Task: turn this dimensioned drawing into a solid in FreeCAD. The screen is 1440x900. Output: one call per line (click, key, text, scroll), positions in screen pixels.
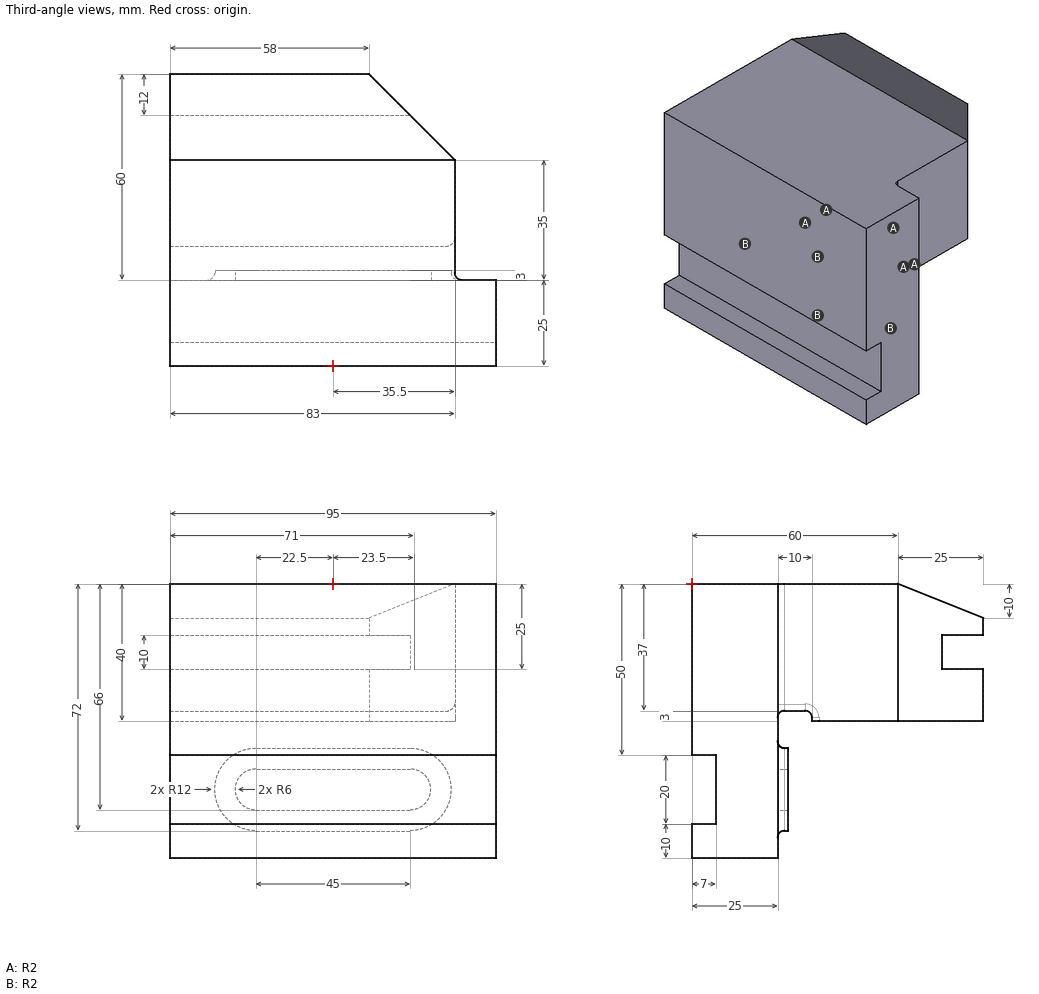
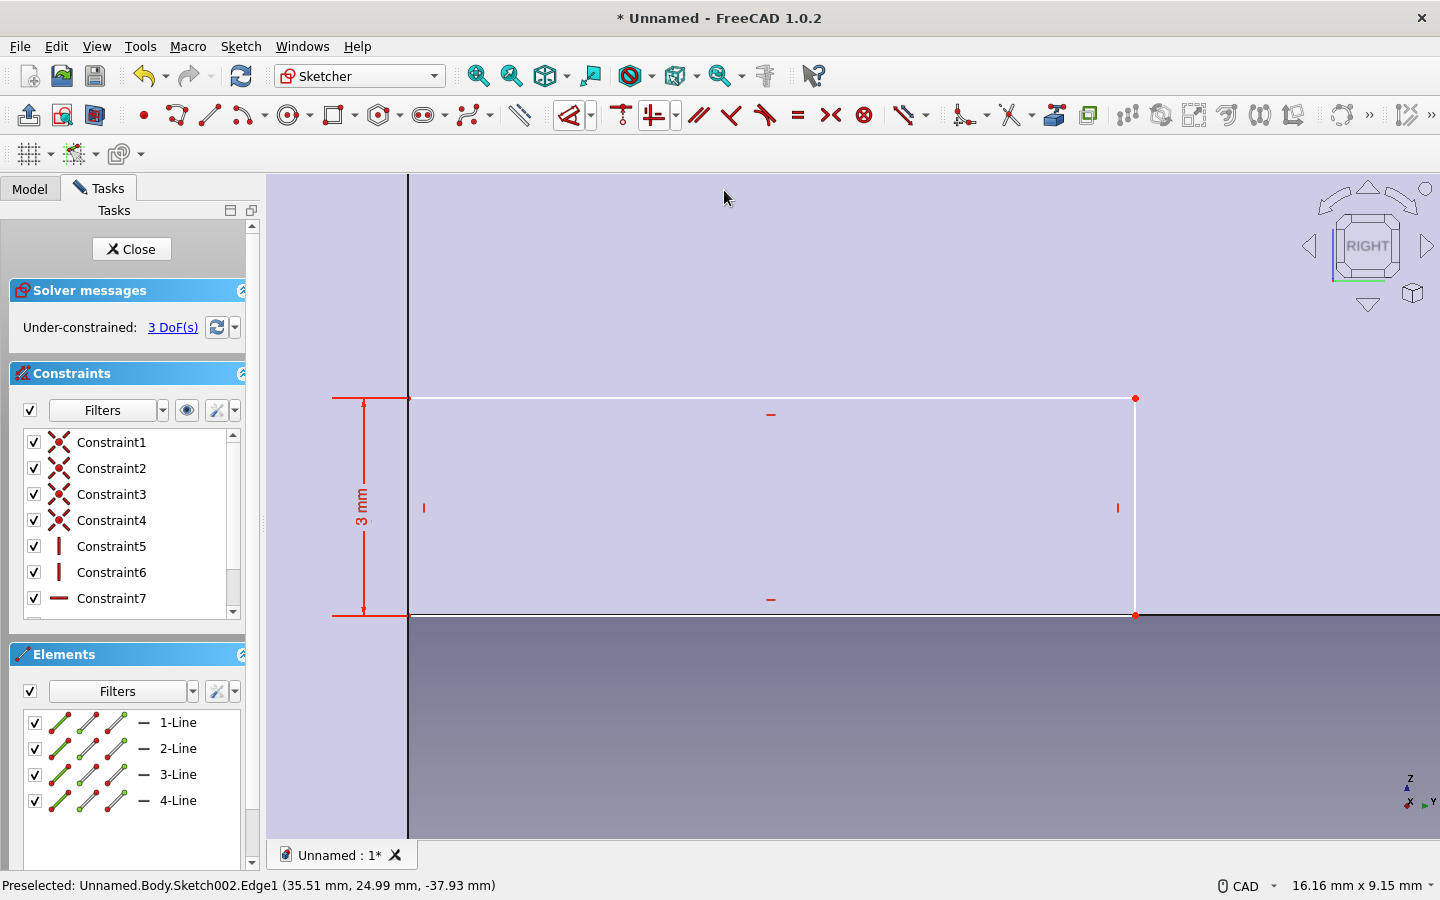
click(626, 616)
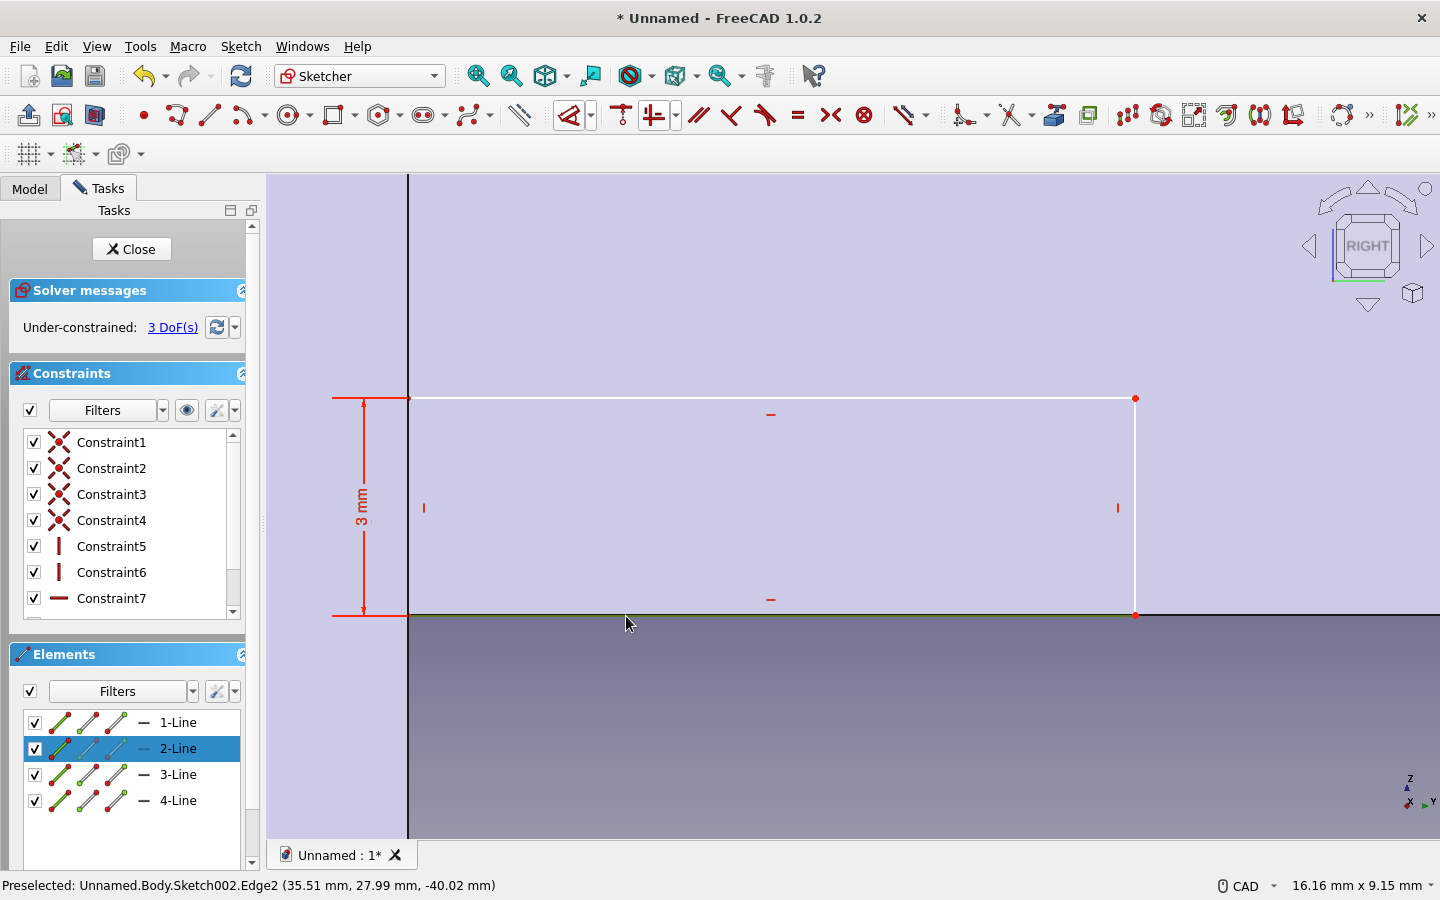
key(l)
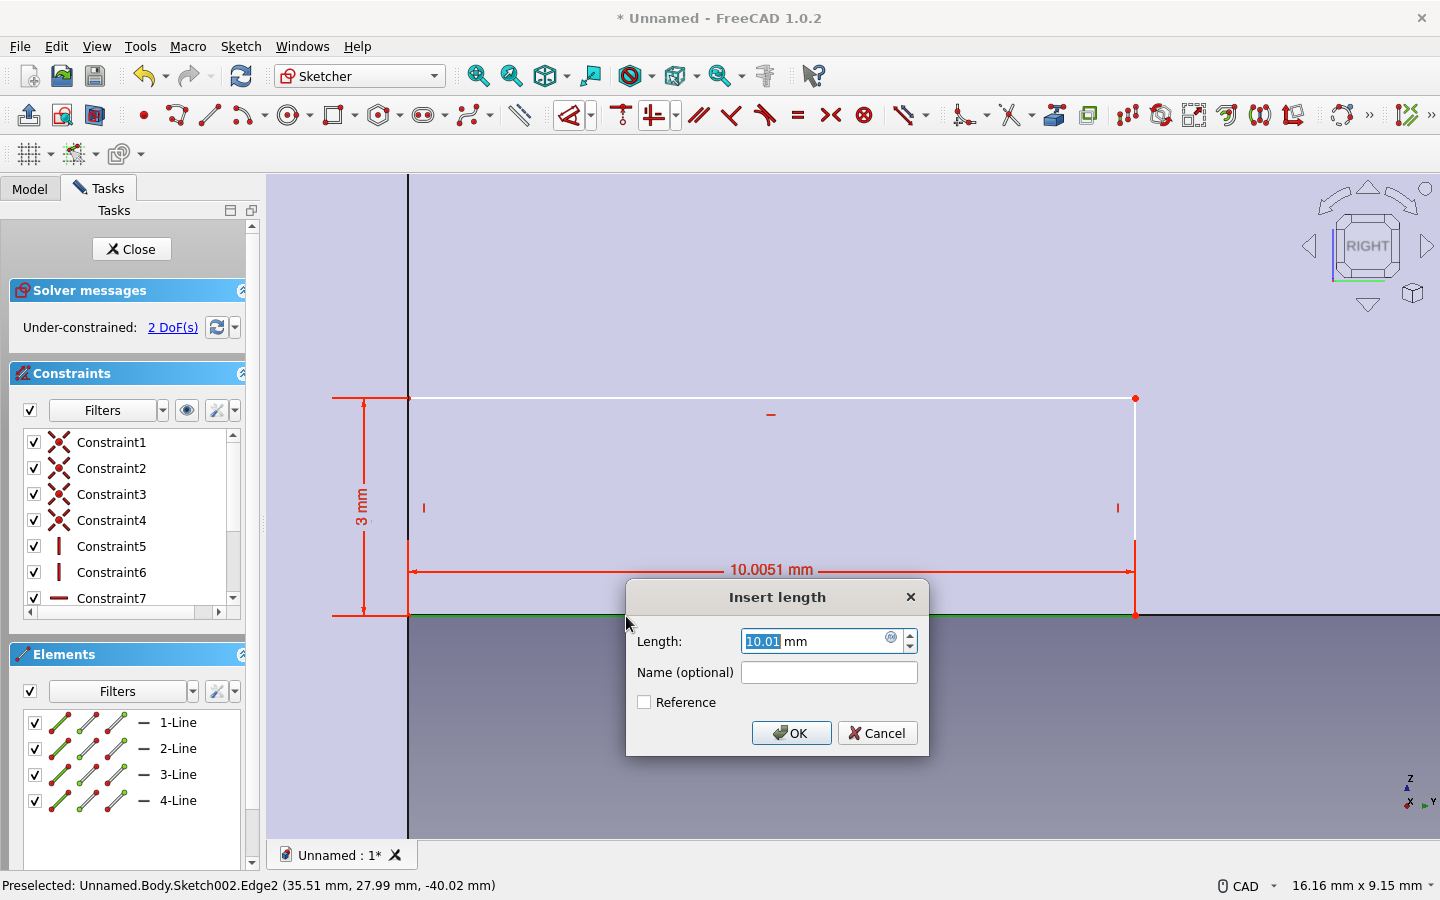
text(10)
key(Return)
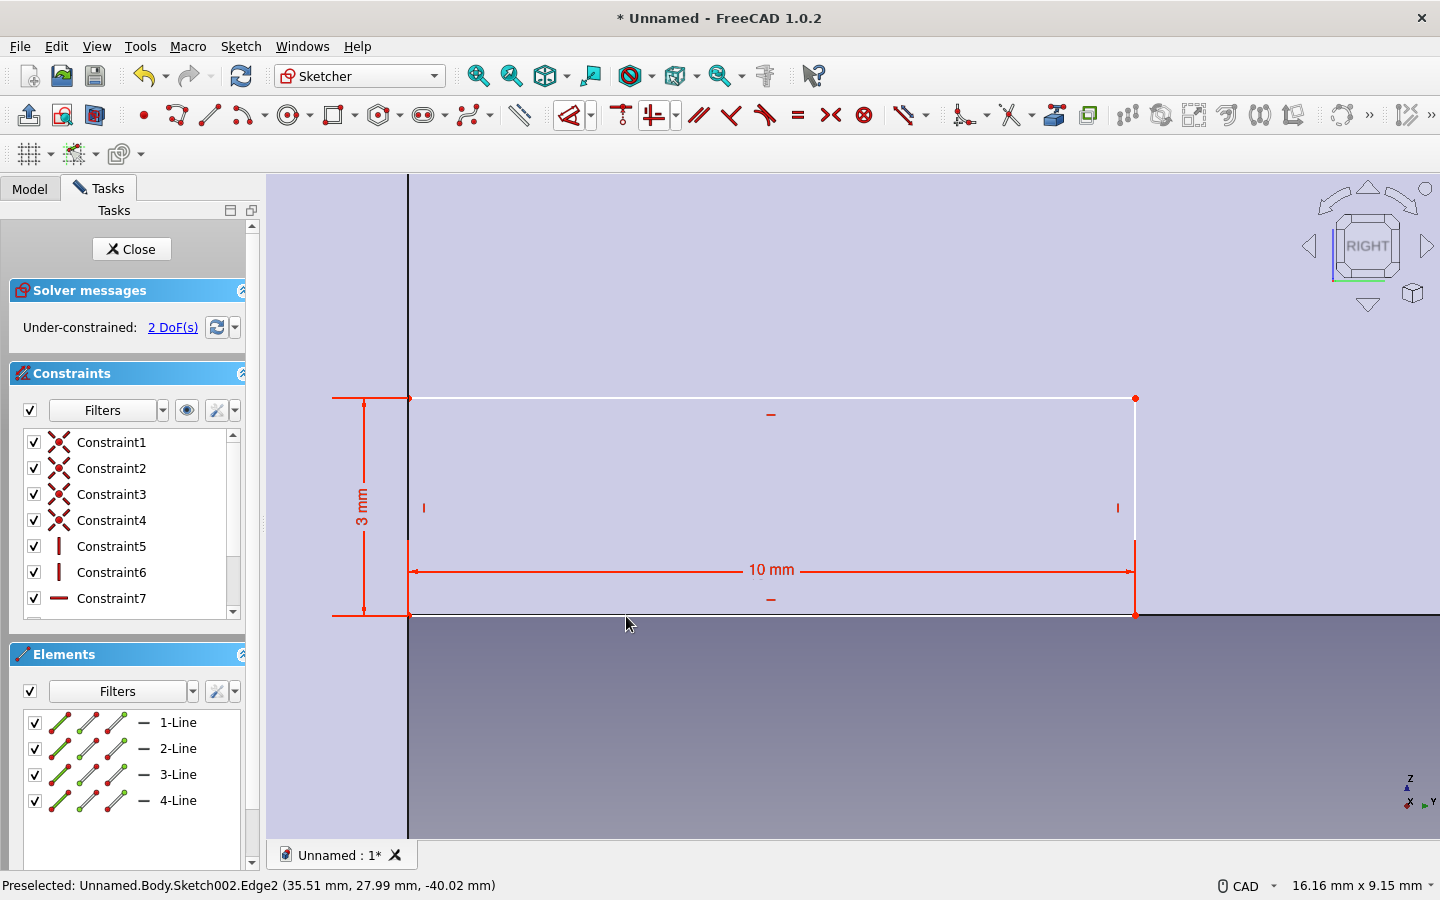
click(408, 398)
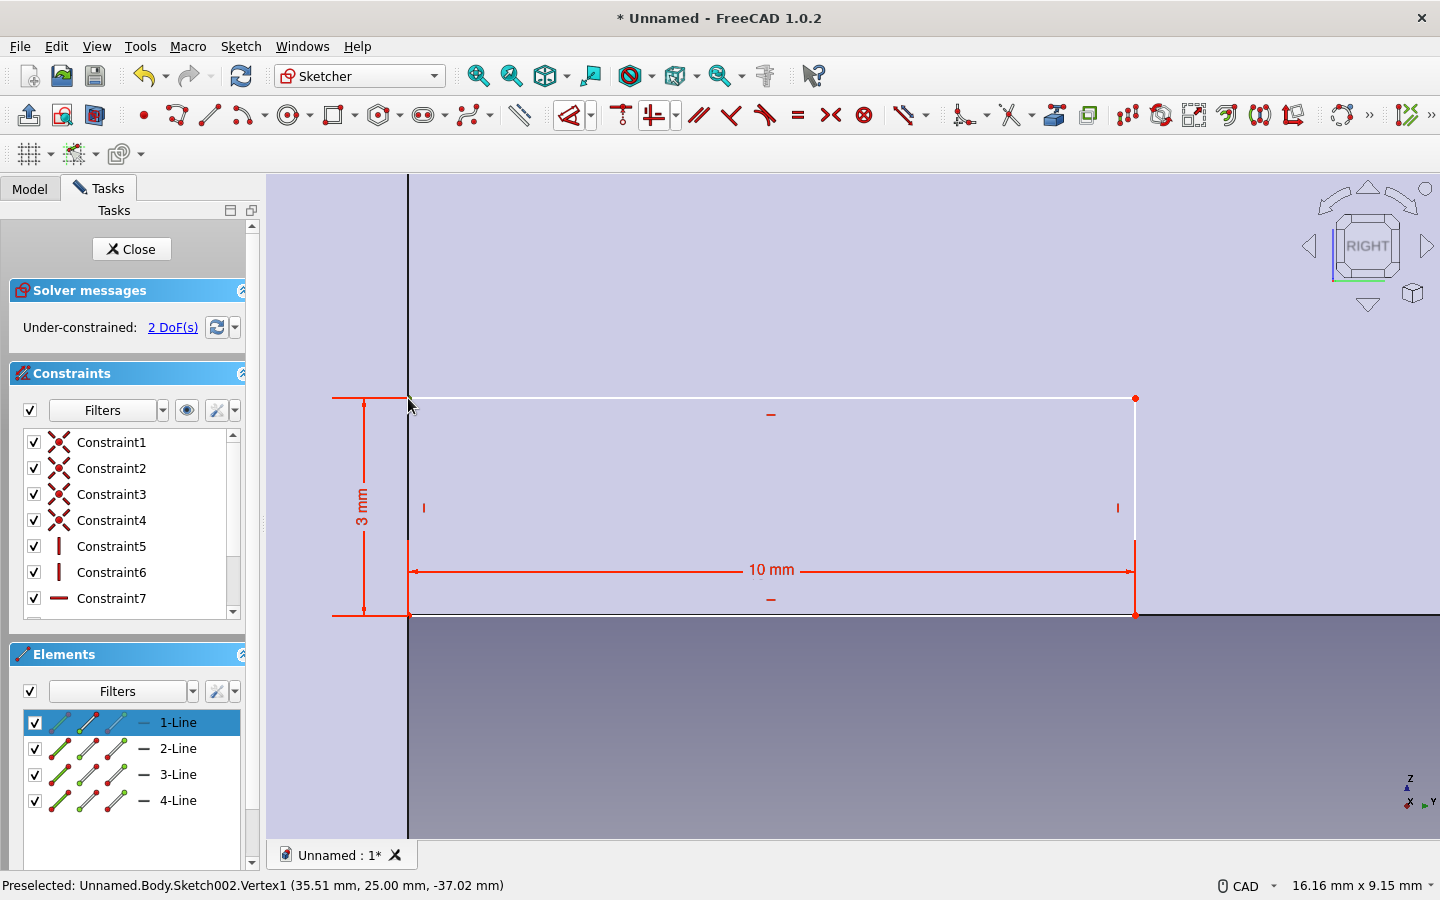
key(l)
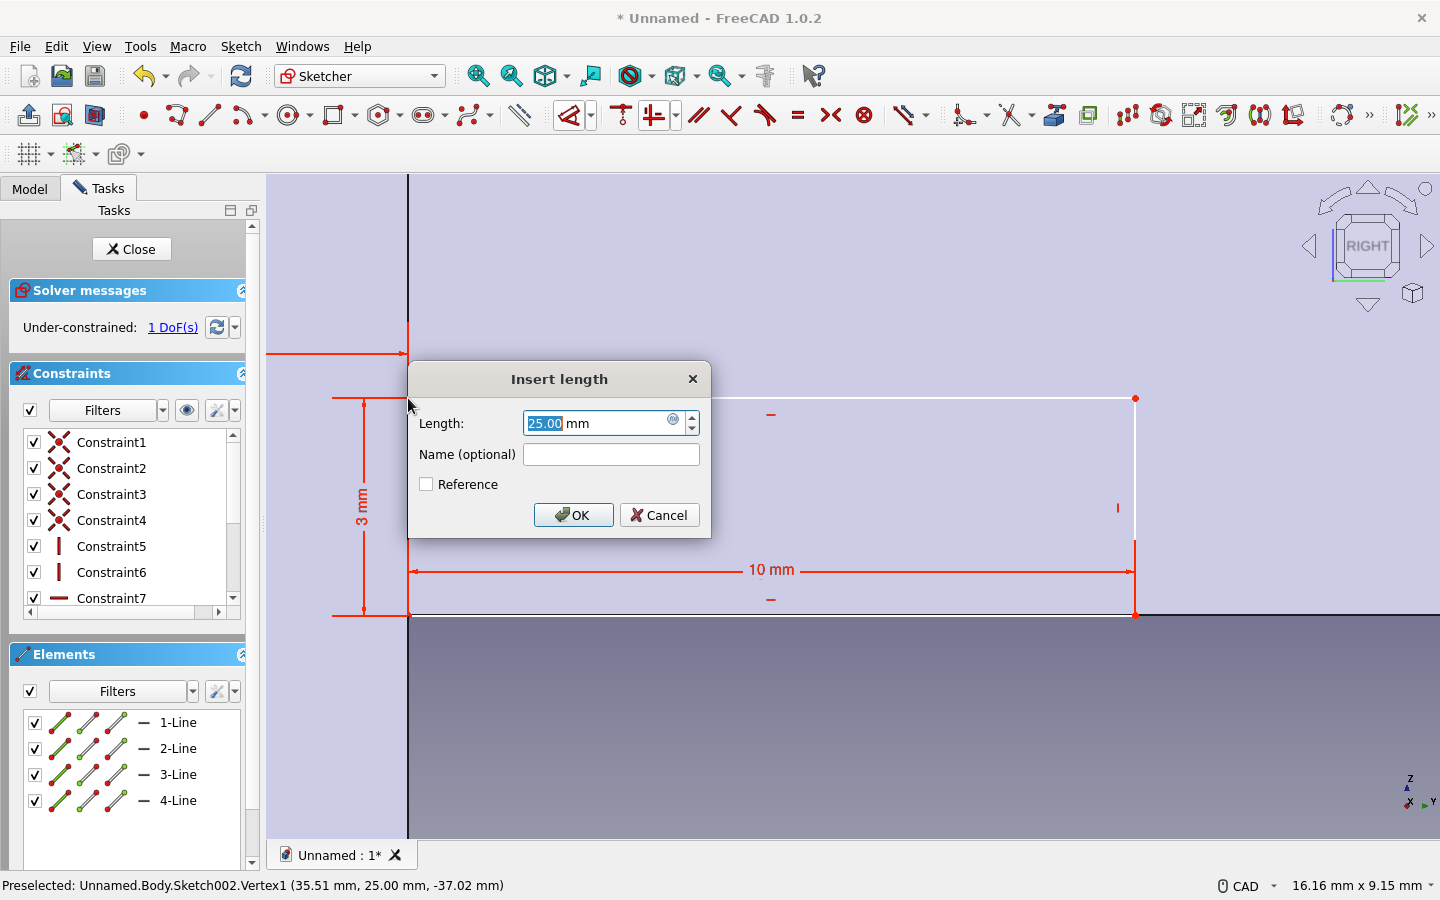
text(25)
key(Return)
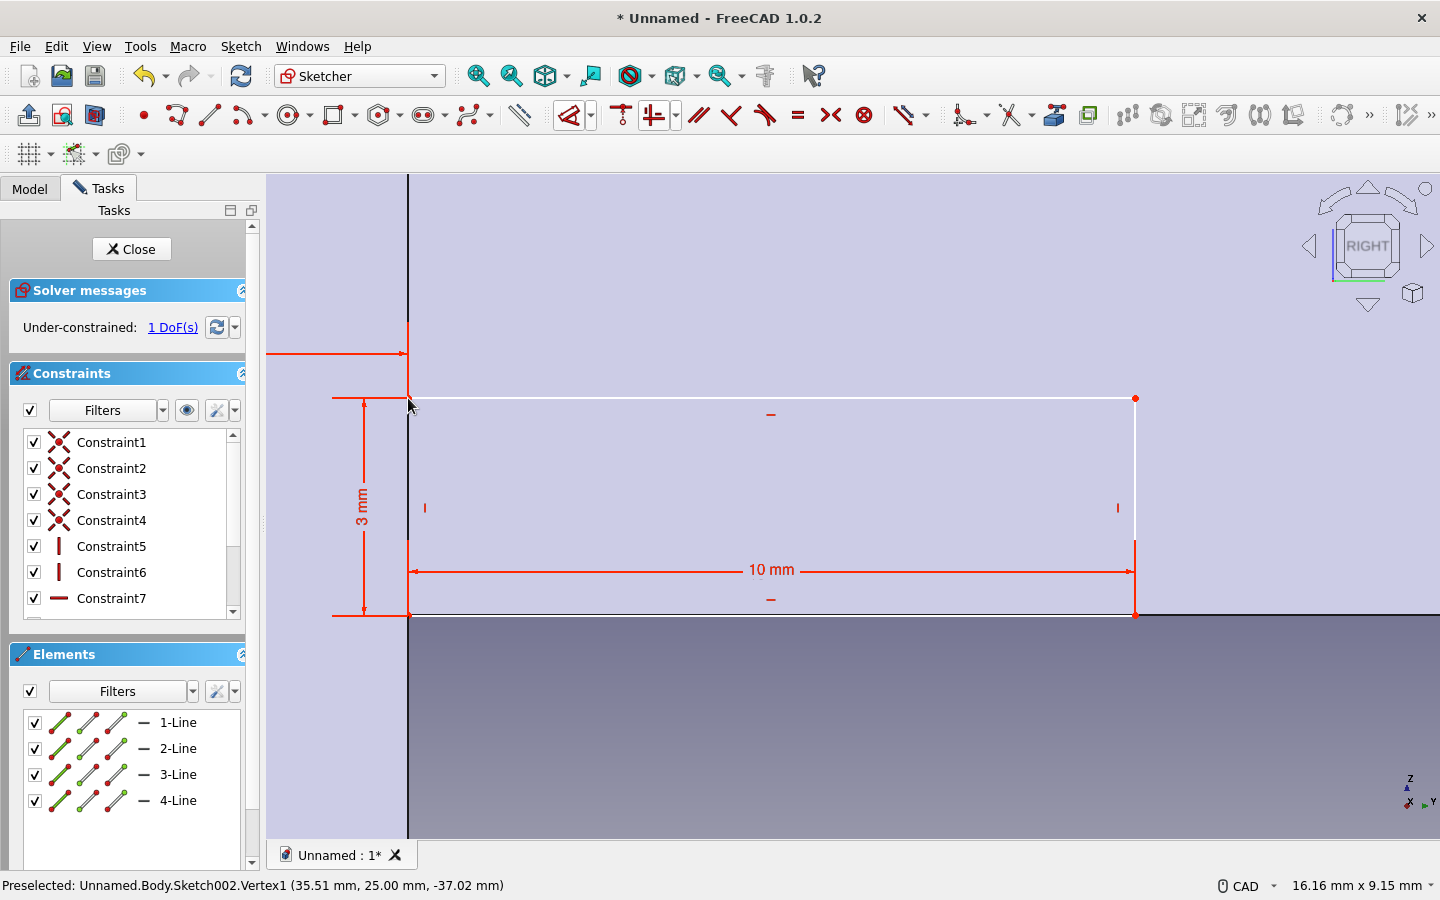
click(408, 398)